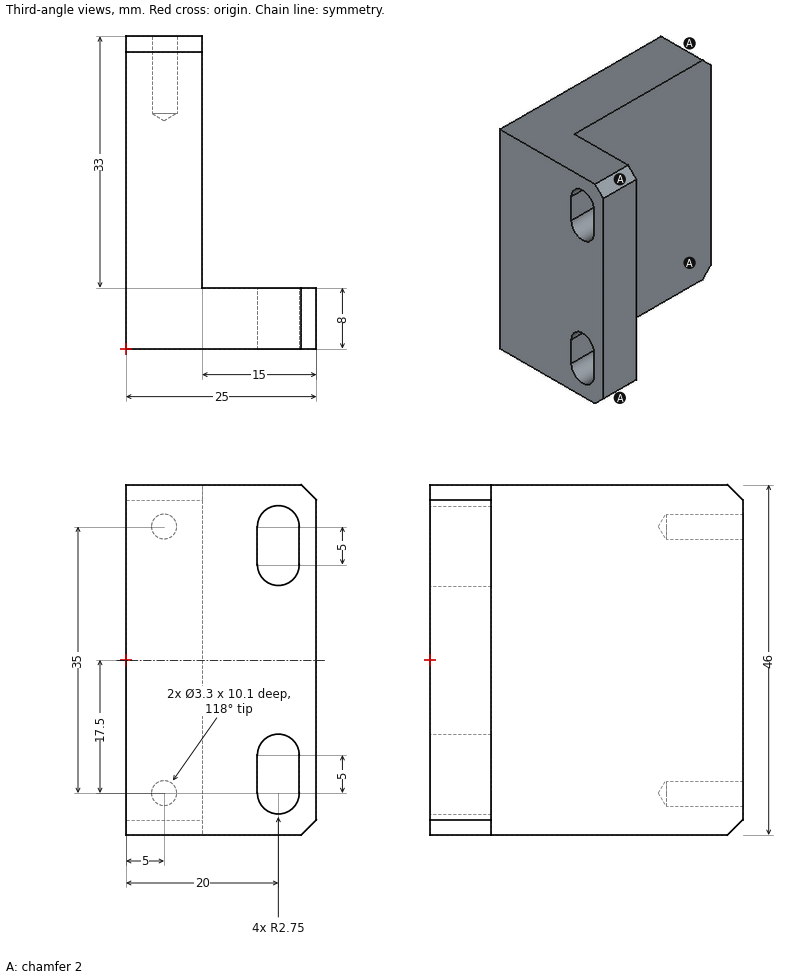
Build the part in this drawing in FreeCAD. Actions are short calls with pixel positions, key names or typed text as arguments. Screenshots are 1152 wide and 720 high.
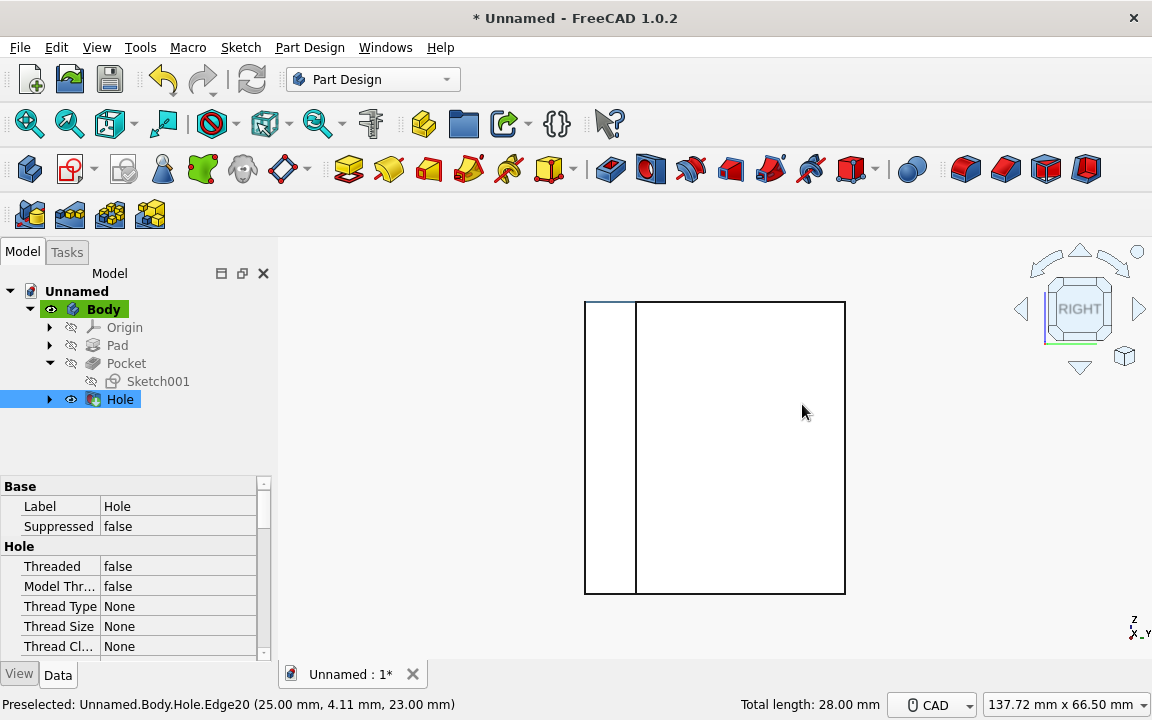
click(610, 593, ctrl)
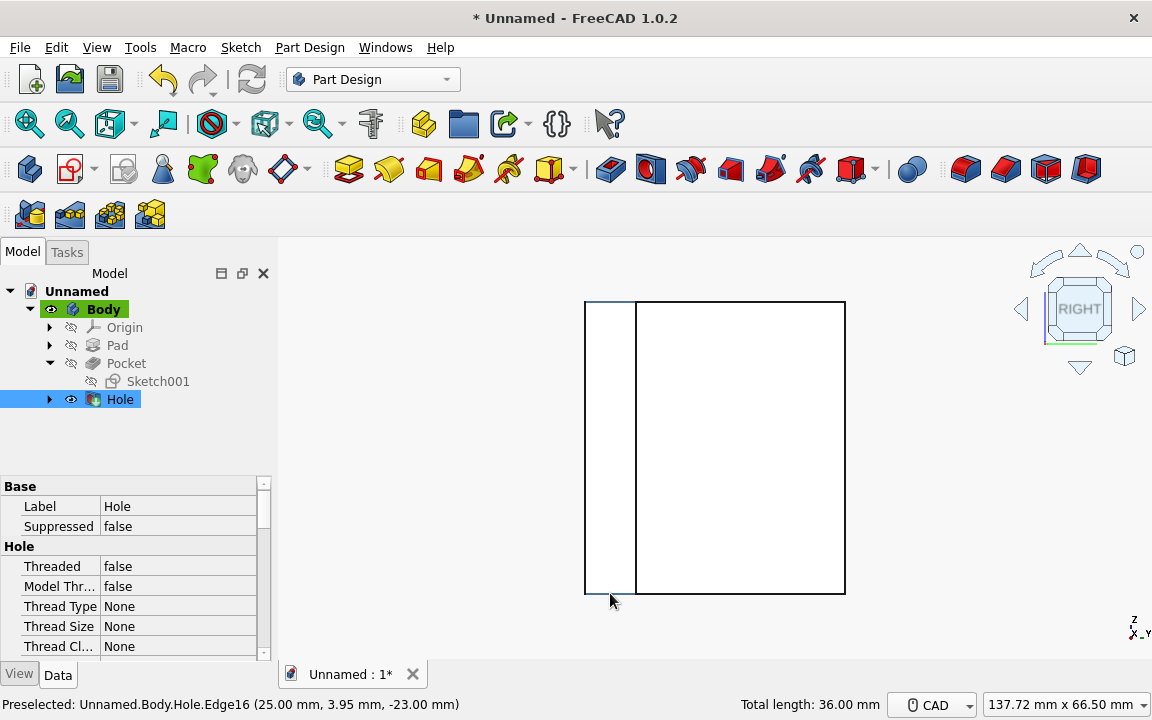
click(1006, 170)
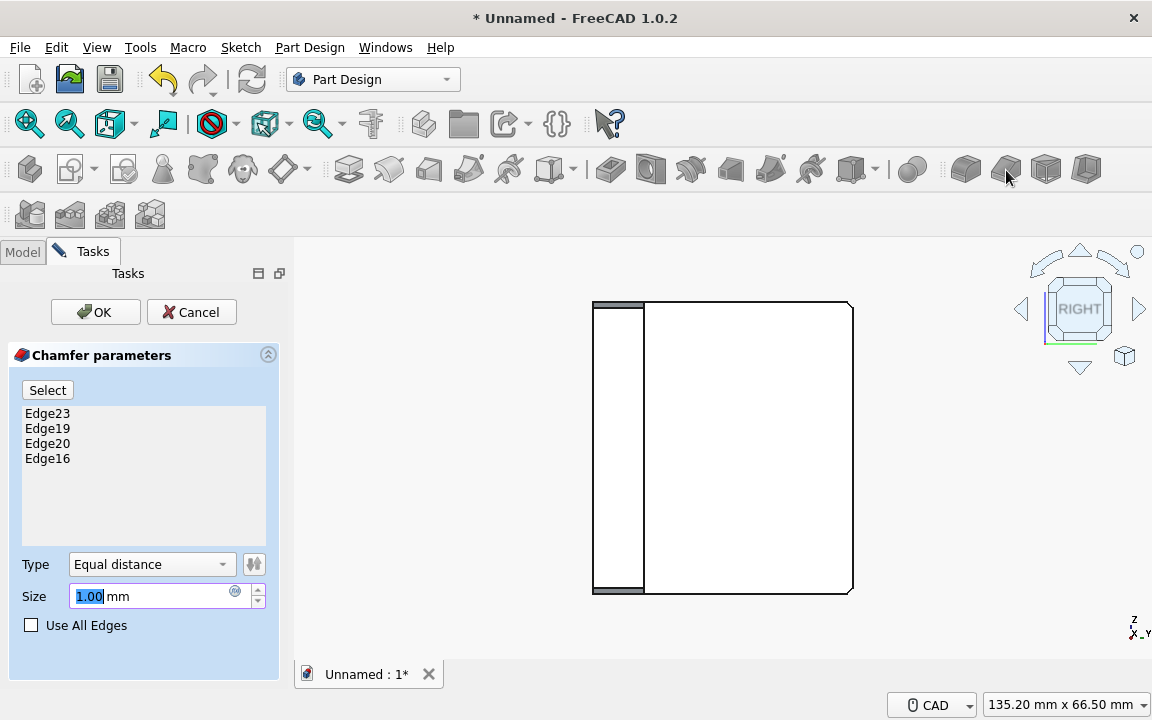
text(2)
key(Tab)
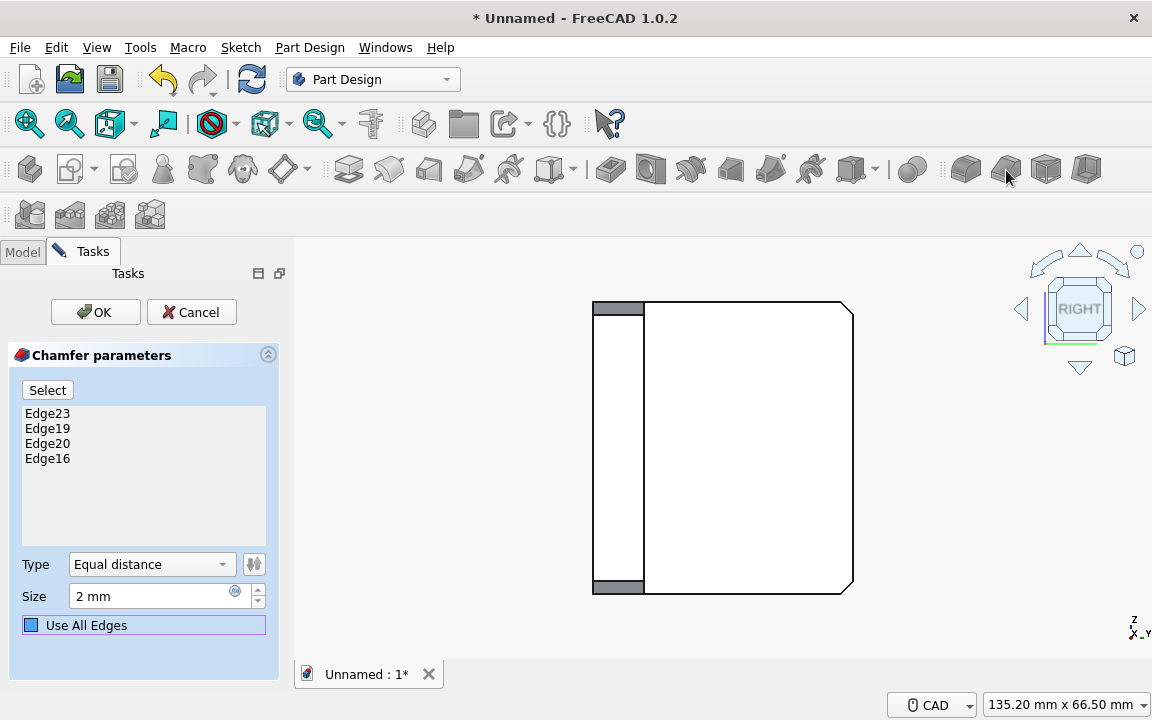
click(96, 312)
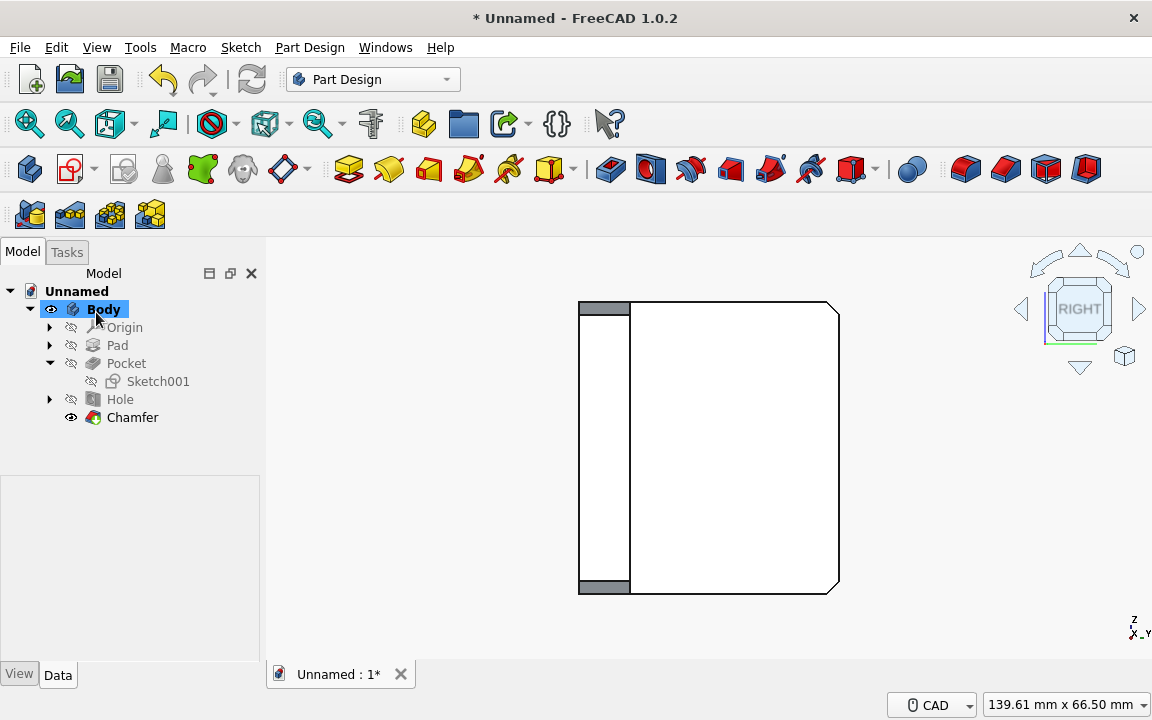
key(0)